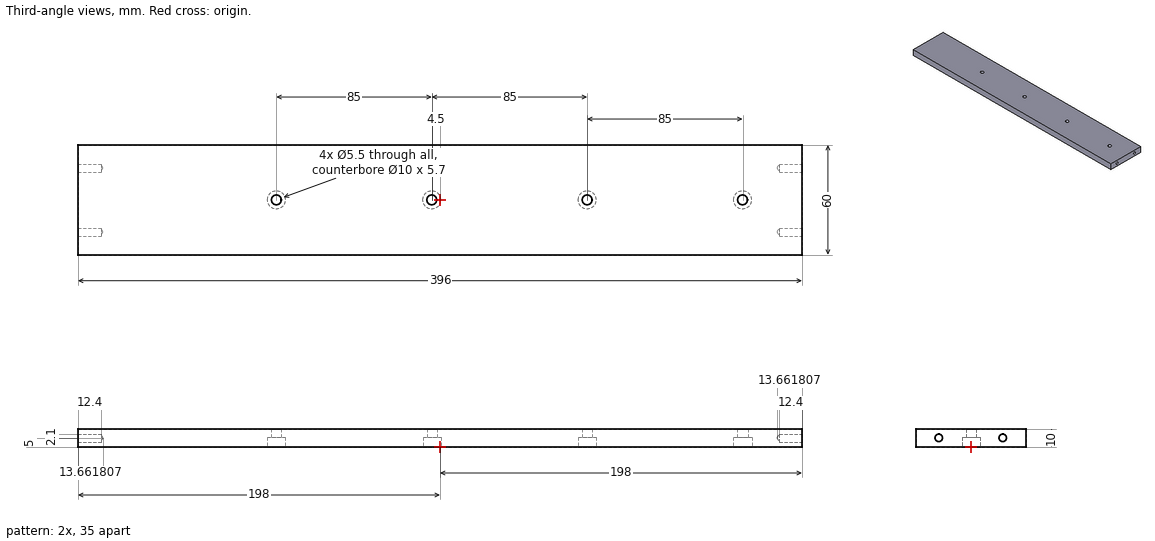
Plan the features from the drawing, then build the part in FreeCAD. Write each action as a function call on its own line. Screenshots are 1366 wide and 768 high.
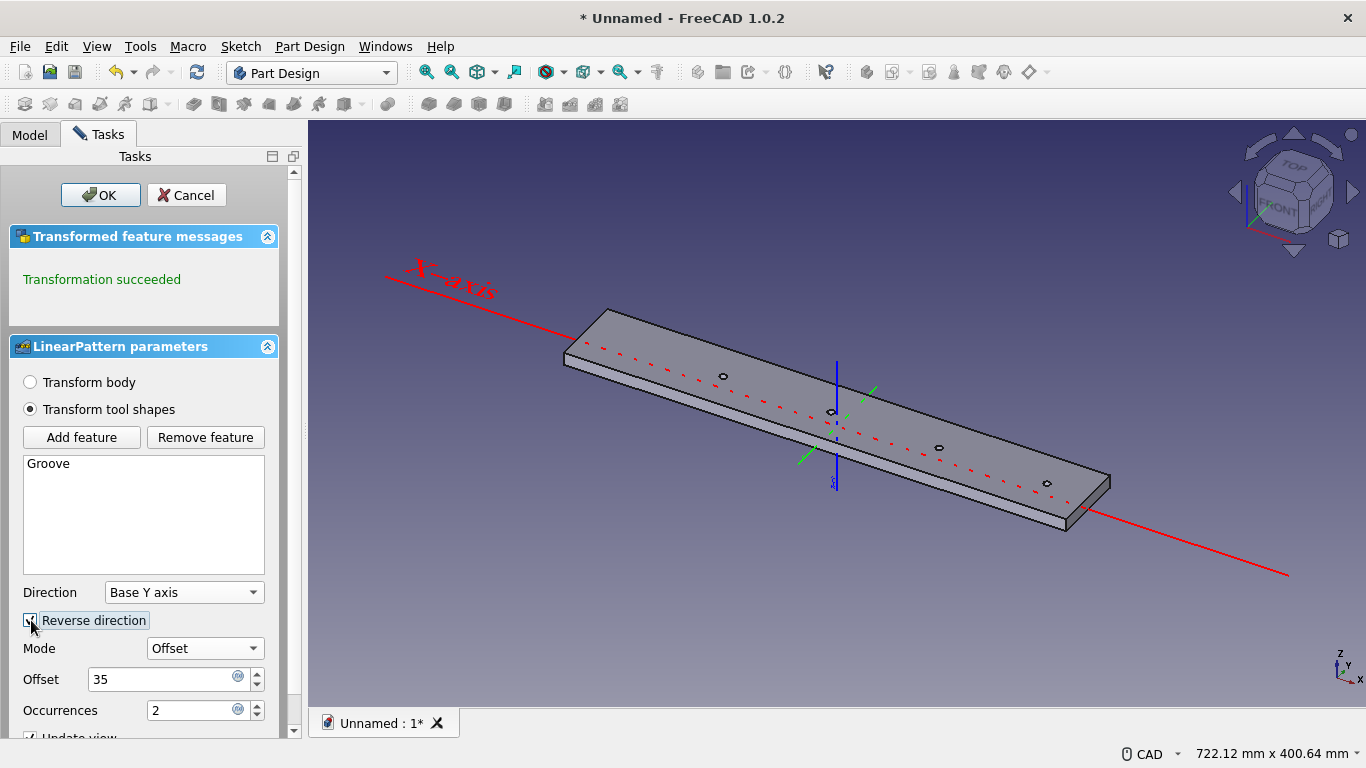
click(101, 195)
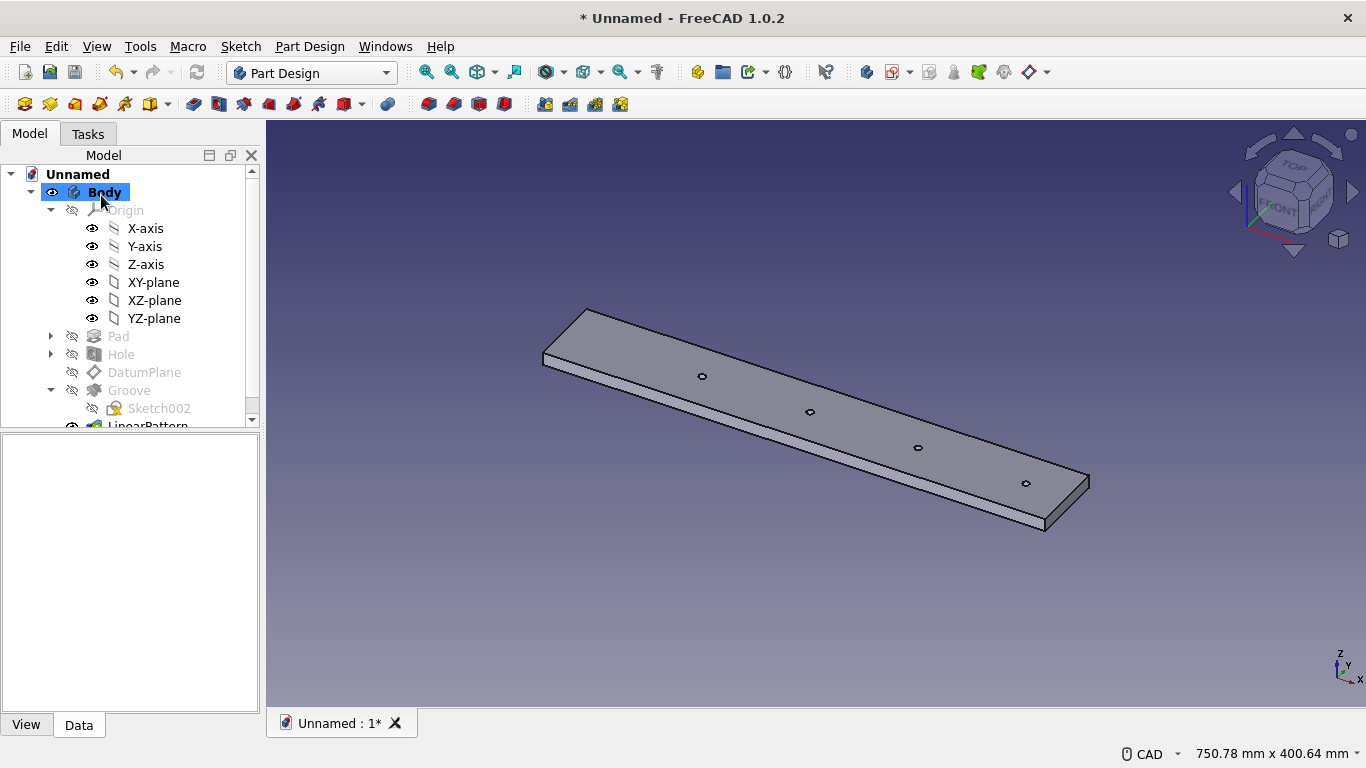
click(117, 390)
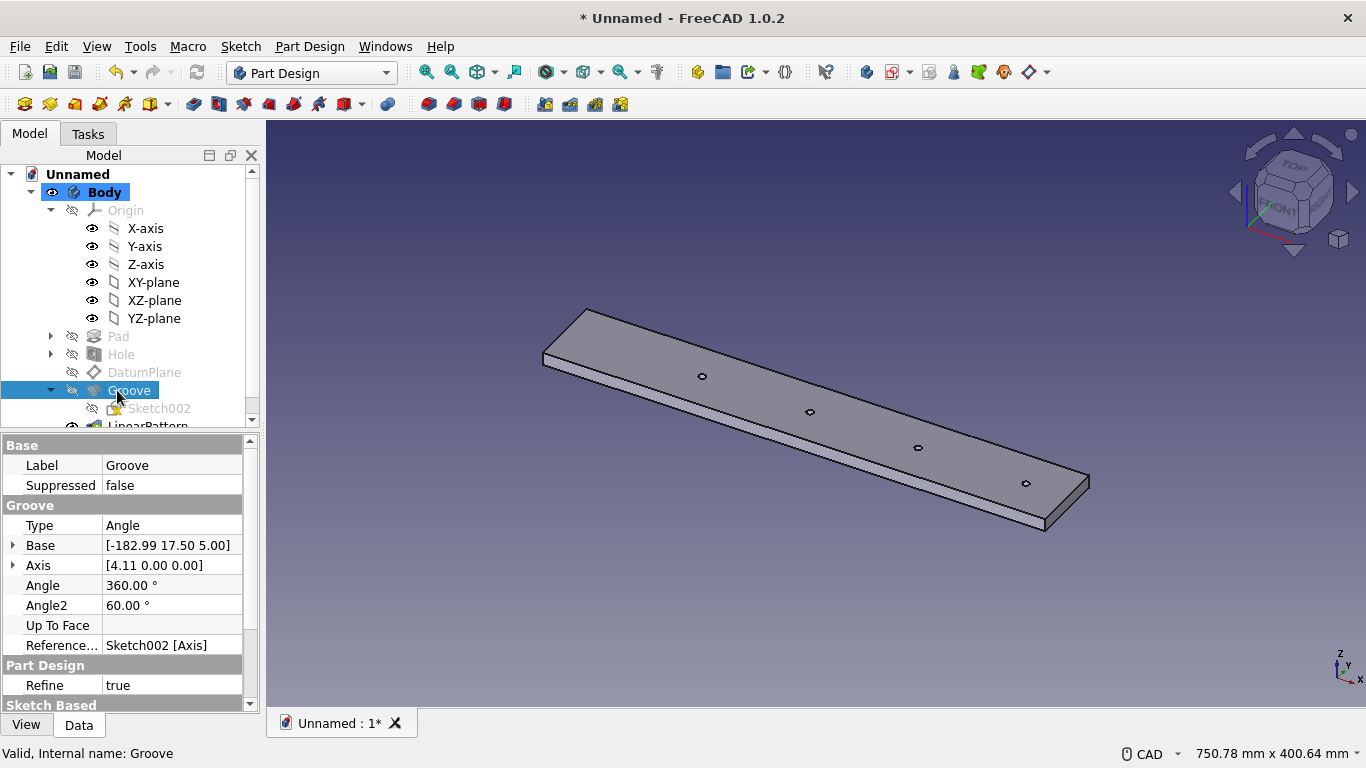
click(545, 104)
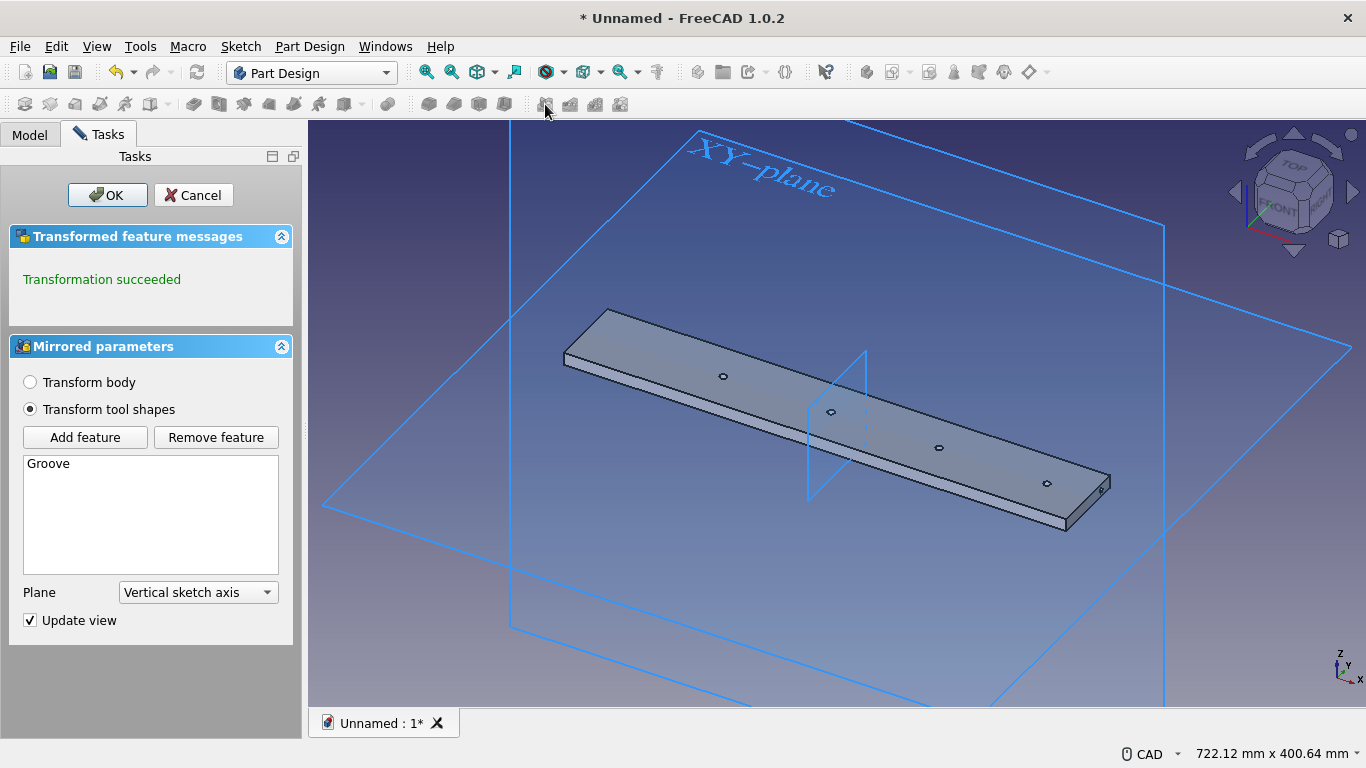
click(199, 592)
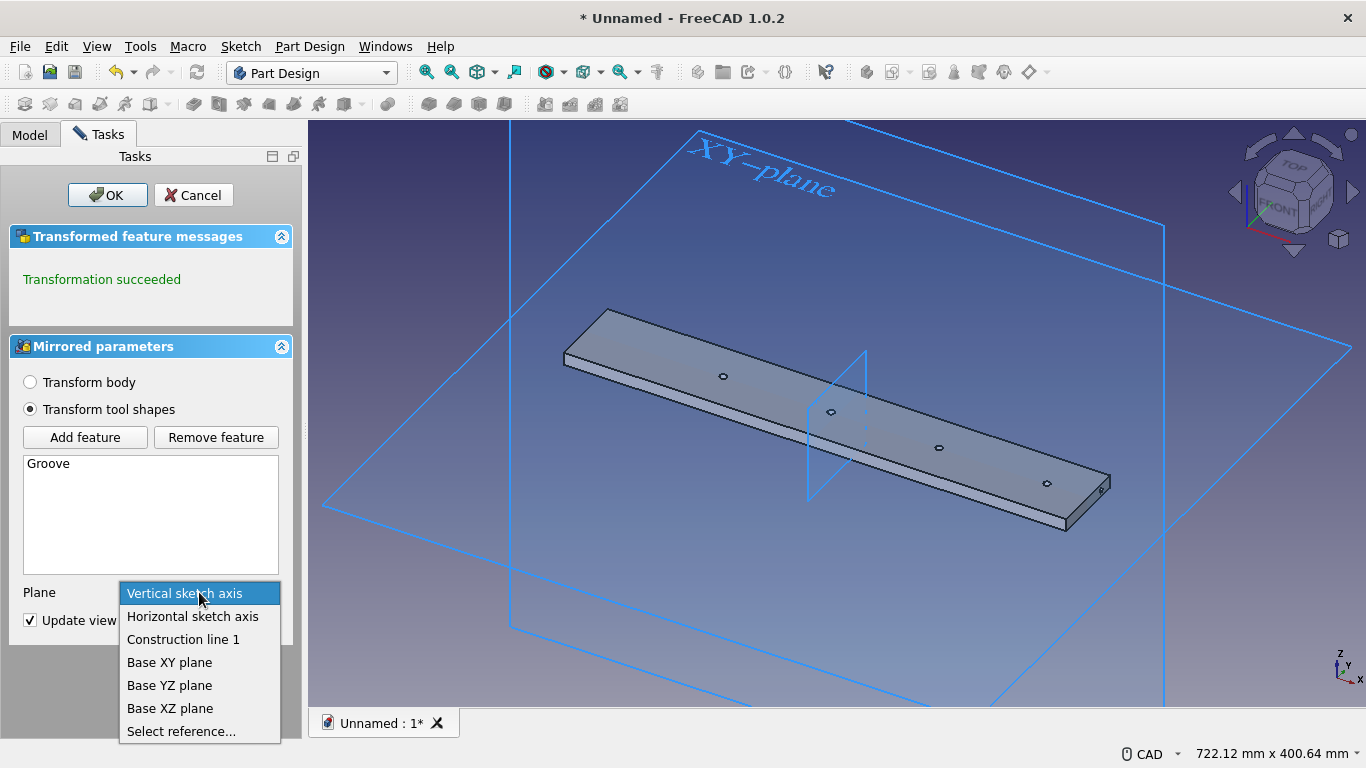
click(198, 686)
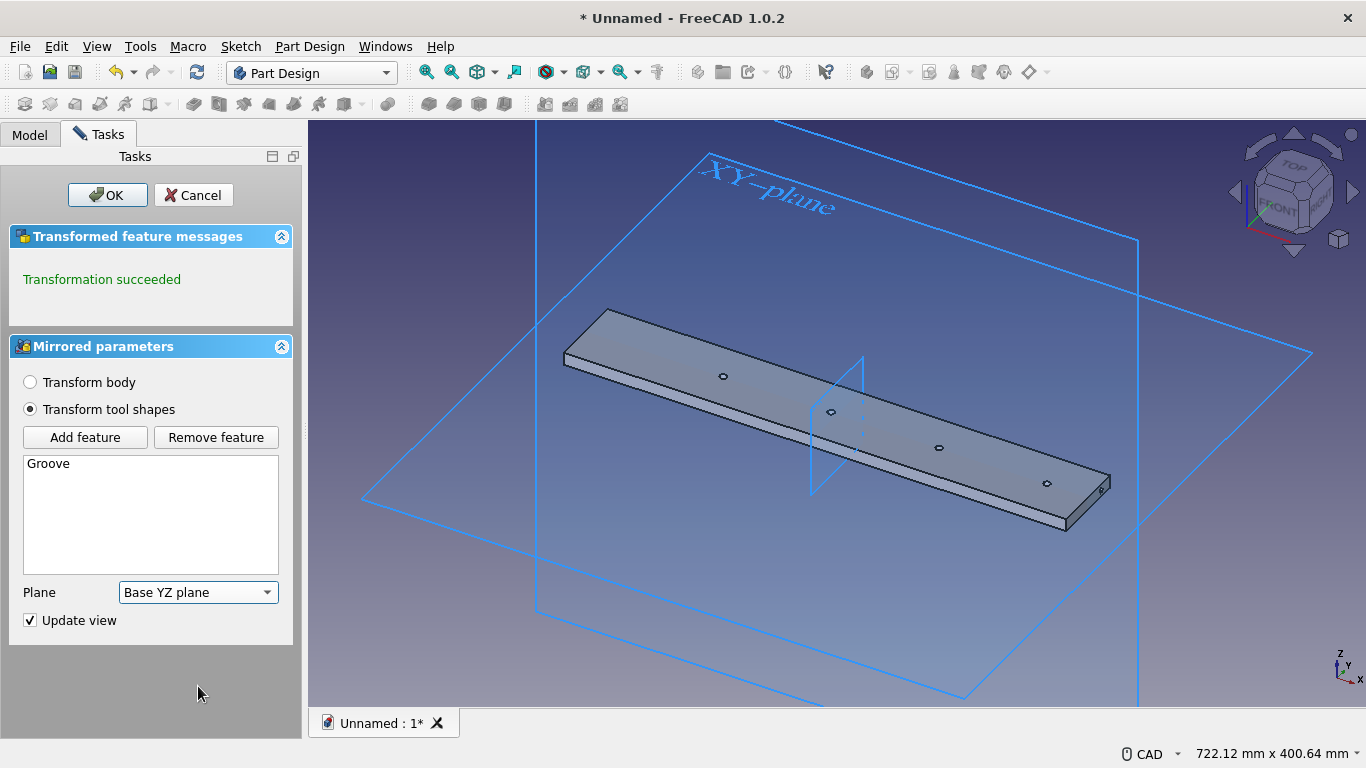
click(108, 195)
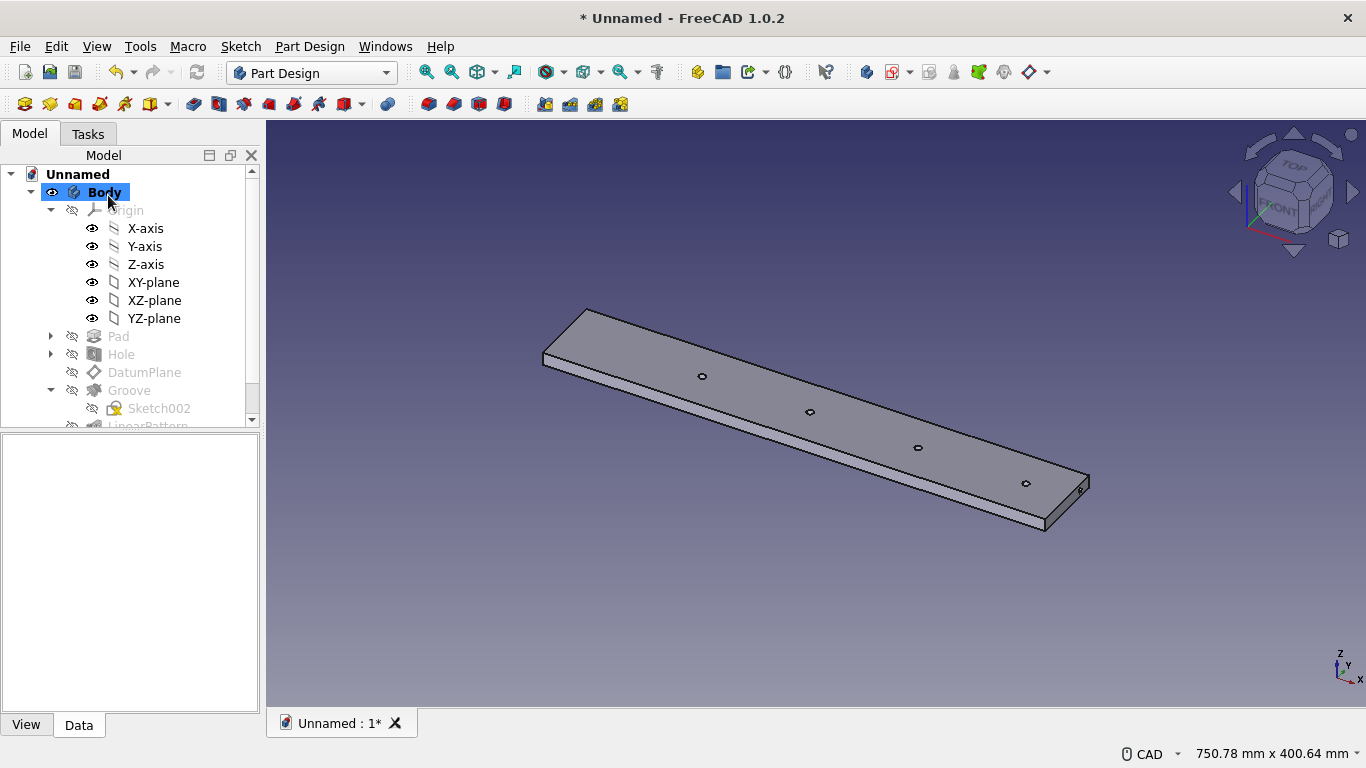
click(137, 300)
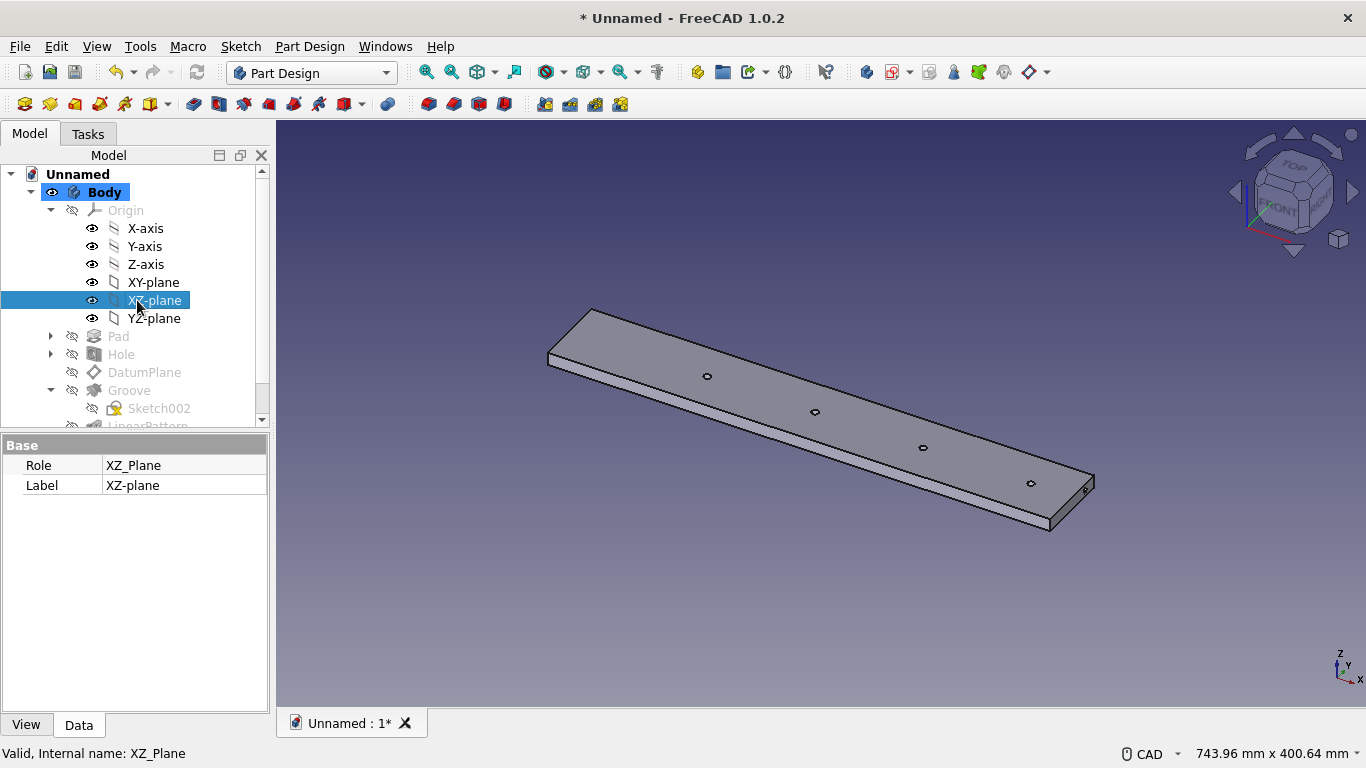
click(1028, 72)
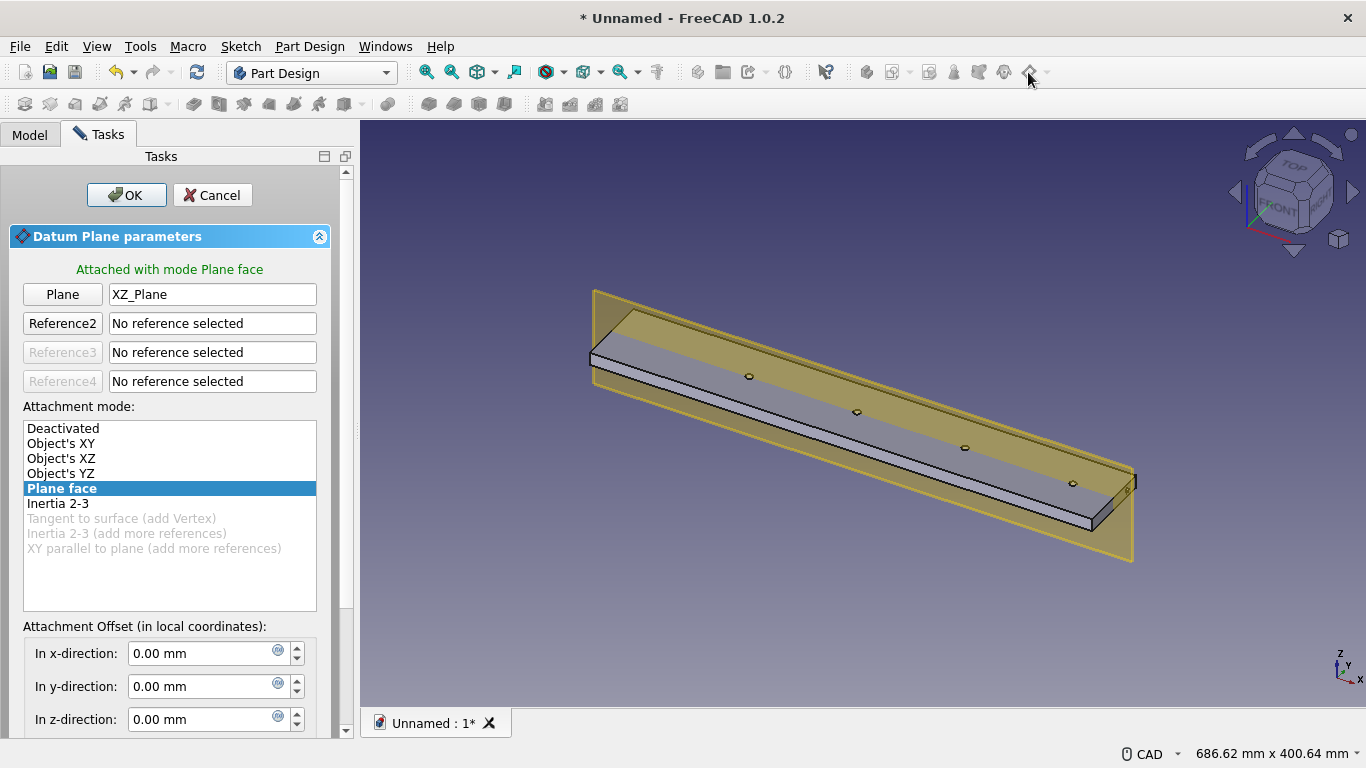
triple_click(210, 720)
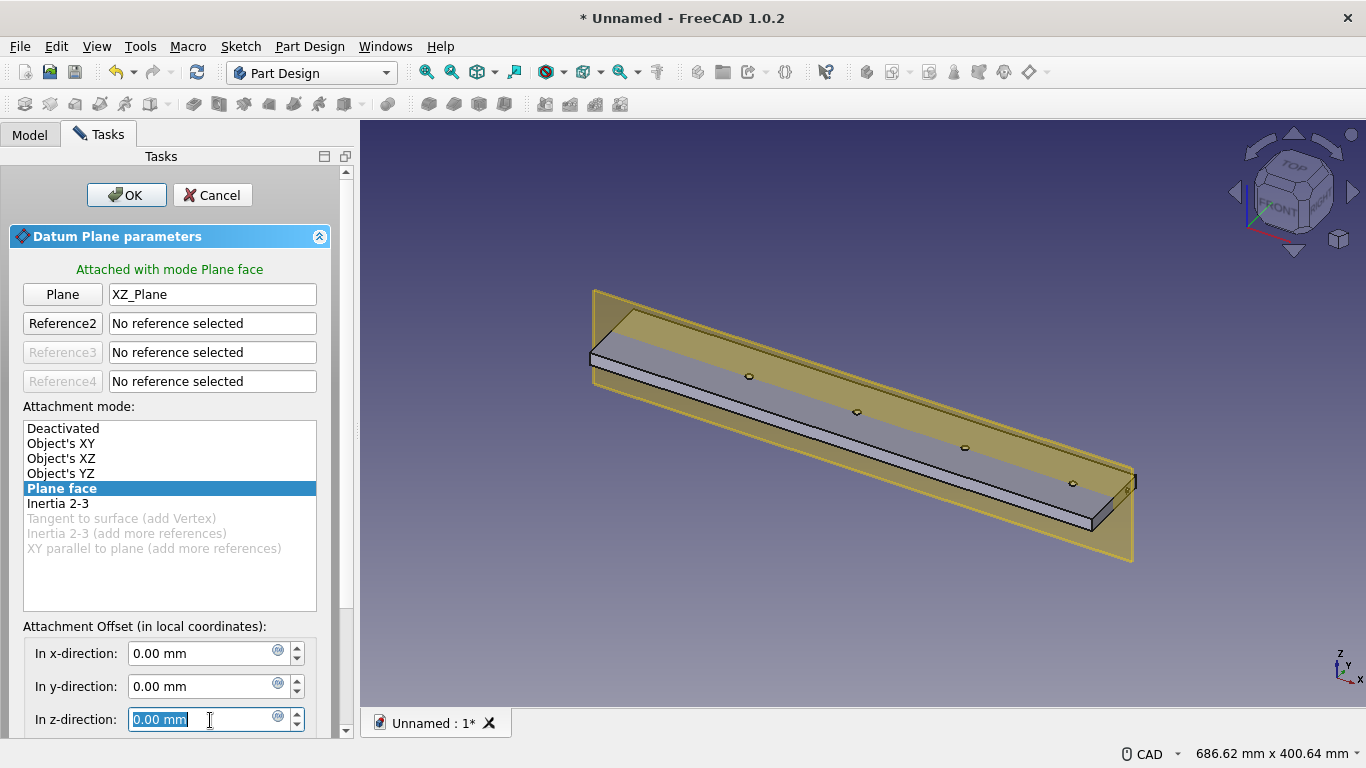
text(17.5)
key(Tab)